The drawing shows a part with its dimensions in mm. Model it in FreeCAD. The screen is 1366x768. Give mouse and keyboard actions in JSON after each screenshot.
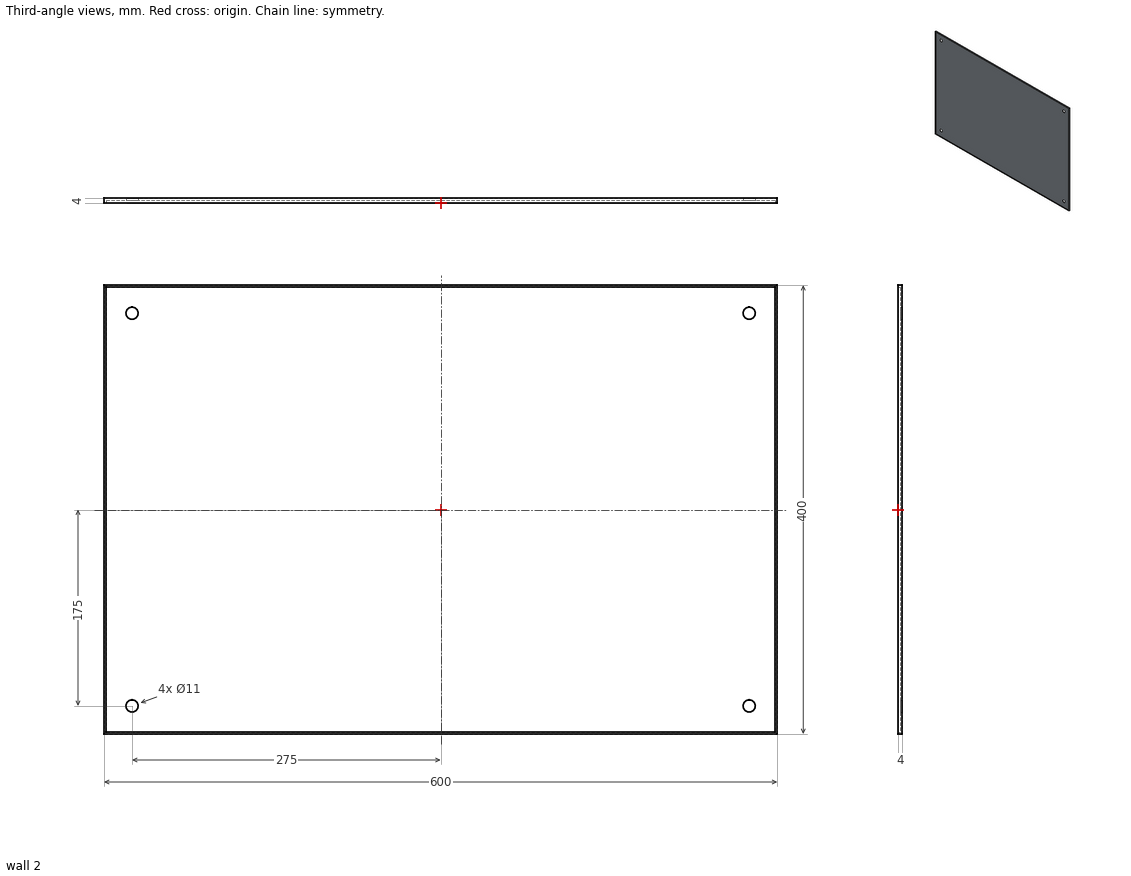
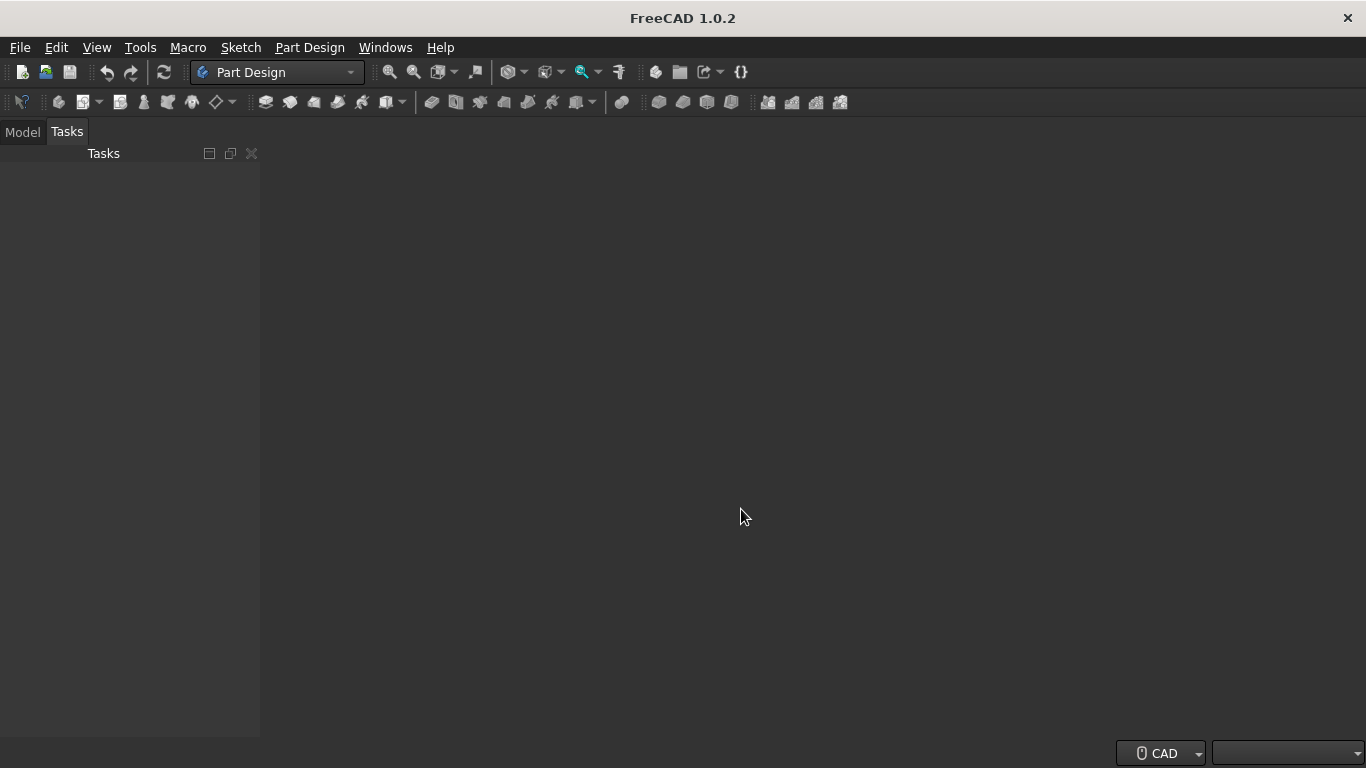
{"action": "key", "text": "ctrl+n"}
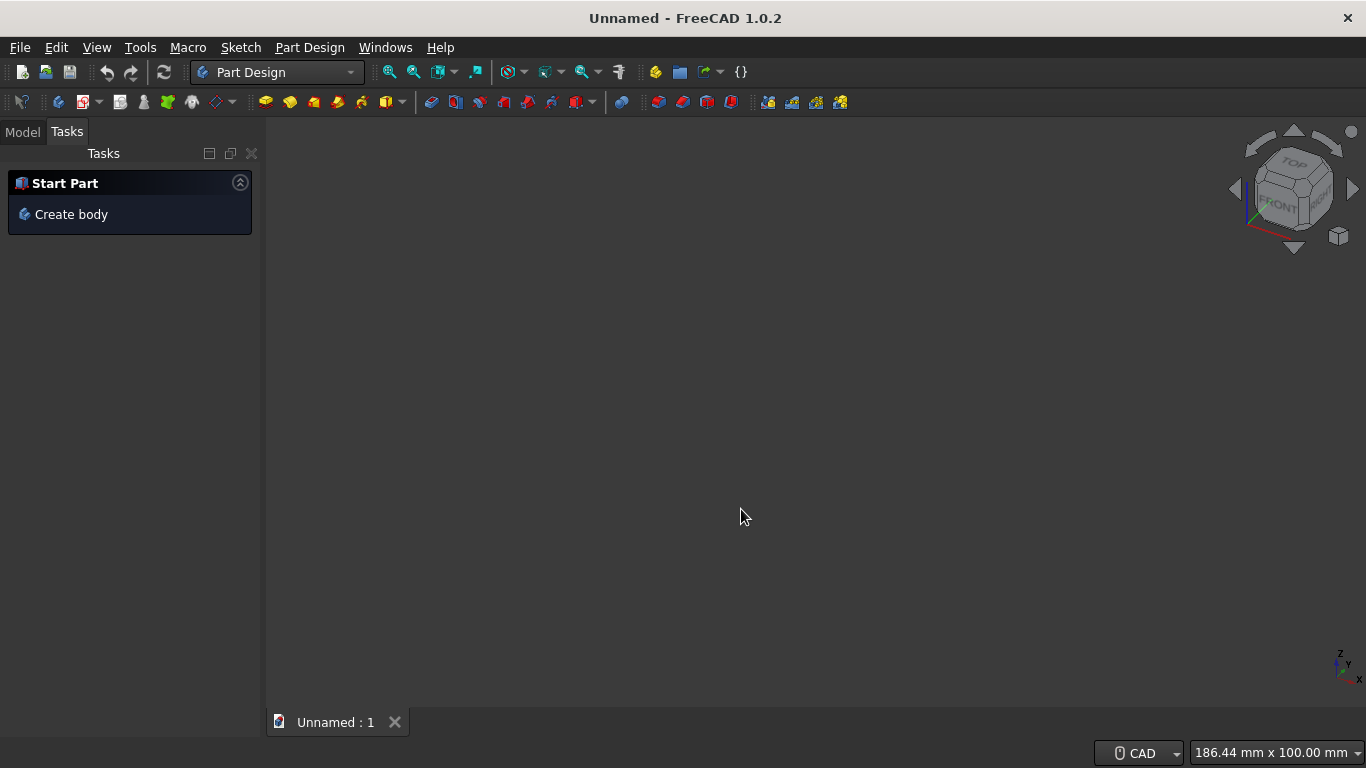
{"action": "left_click", "coordinate": [84, 102]}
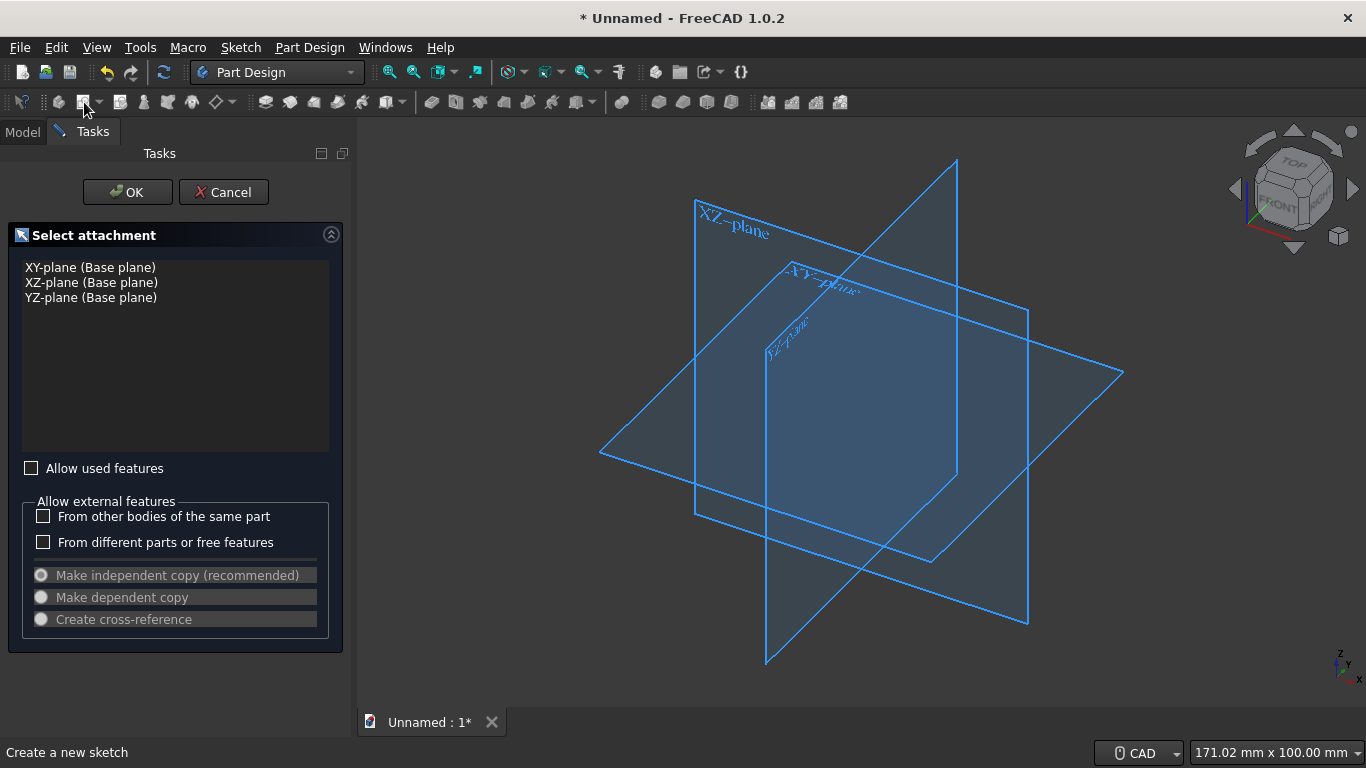
{"action": "left_click", "coordinate": [82, 282]}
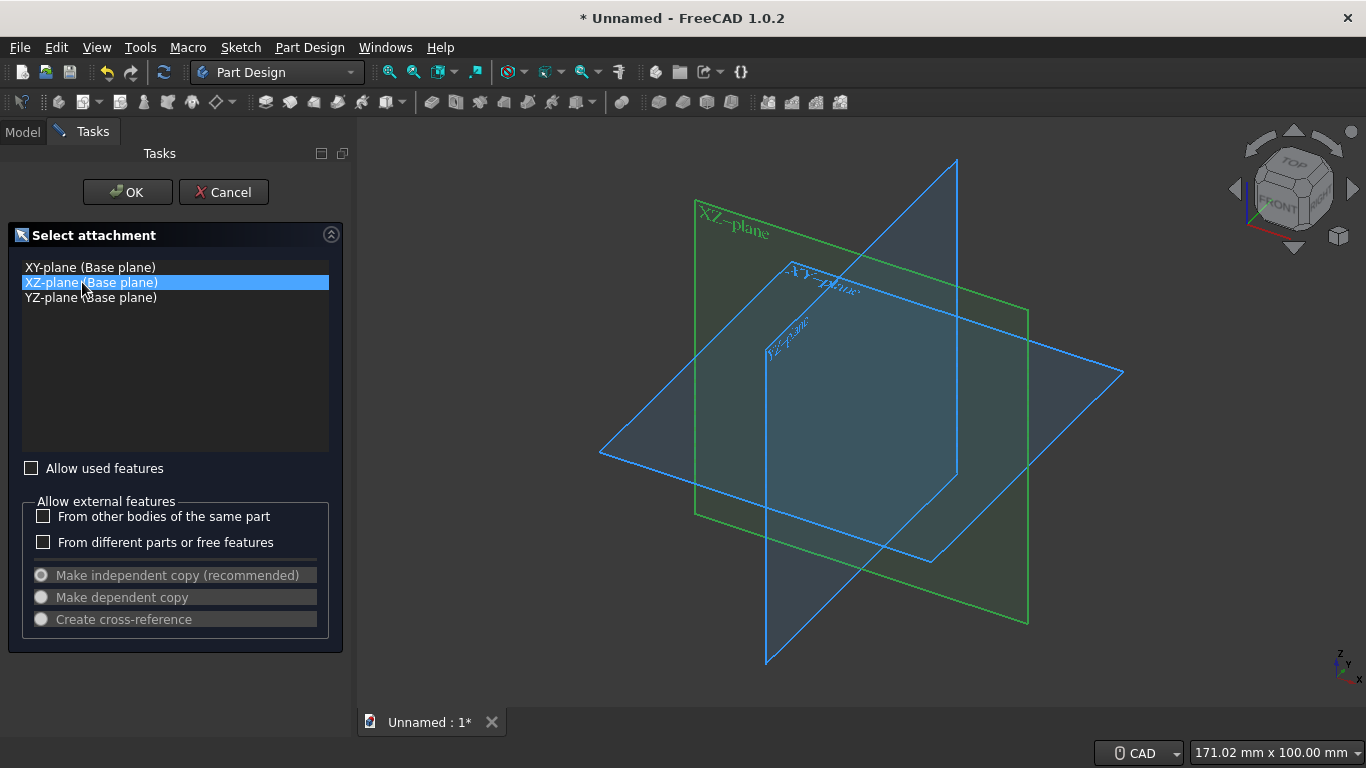
{"action": "left_click", "coordinate": [128, 192]}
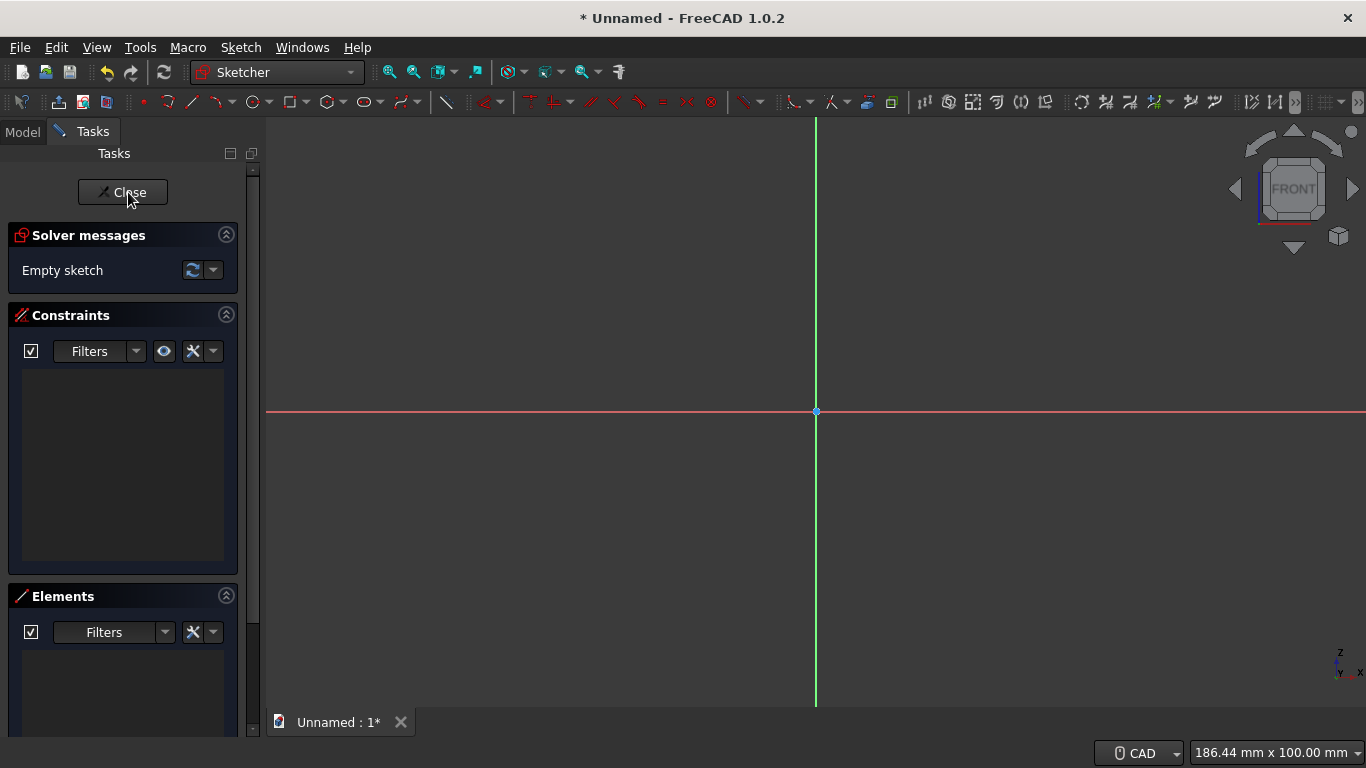
{"action": "scroll", "coordinate": [734, 412], "scroll_direction": "down", "scroll_amount": 9}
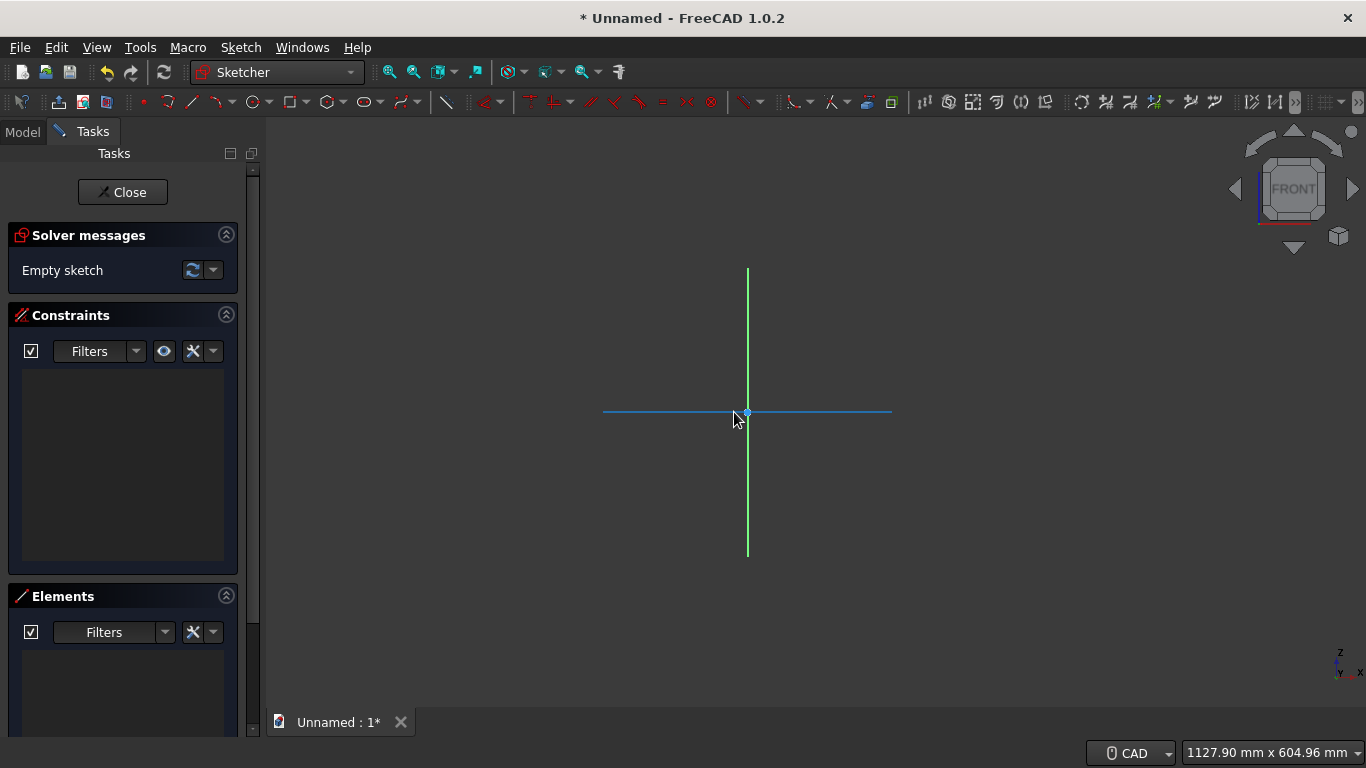
{"action": "key", "text": "g v"}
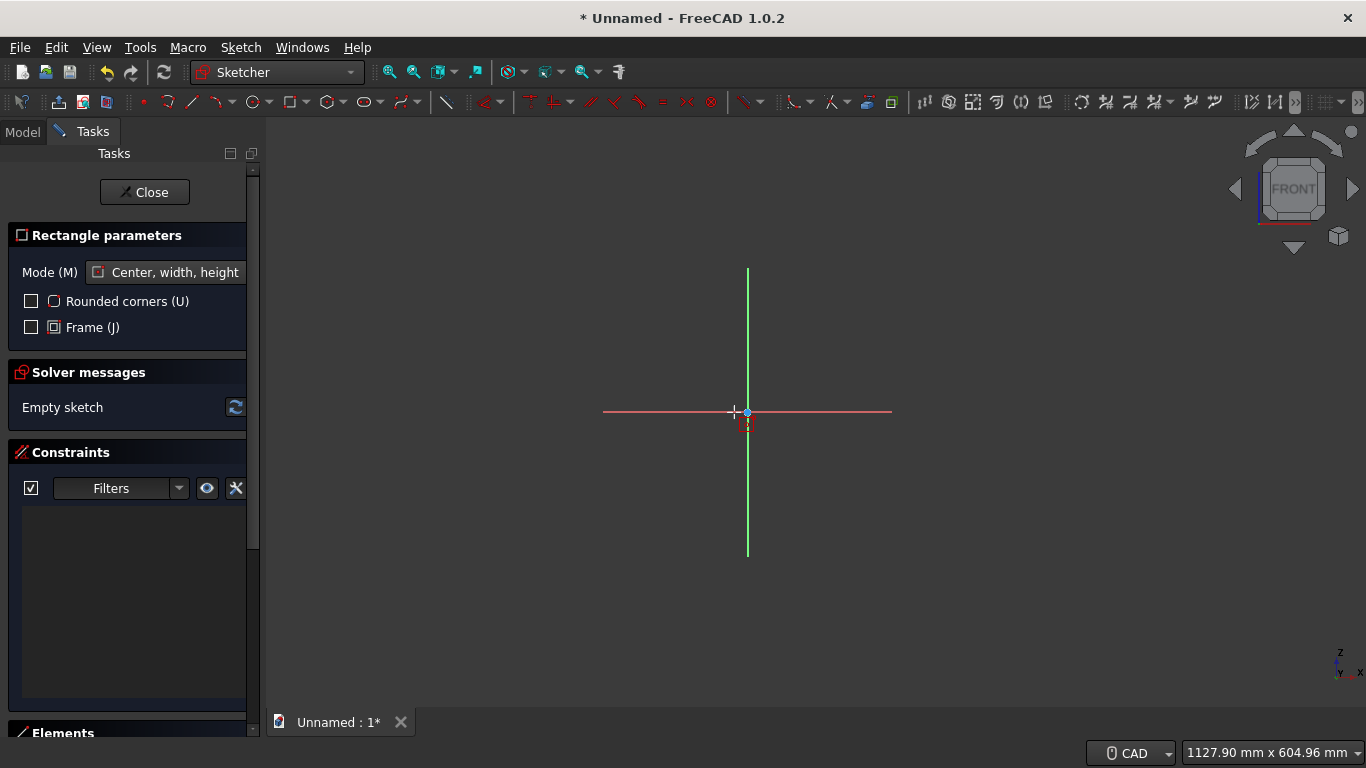
{"action": "left_click", "coordinate": [748, 412]}
{"action": "left_click", "coordinate": [1040, 217]}
{"action": "key", "text": "Escape"}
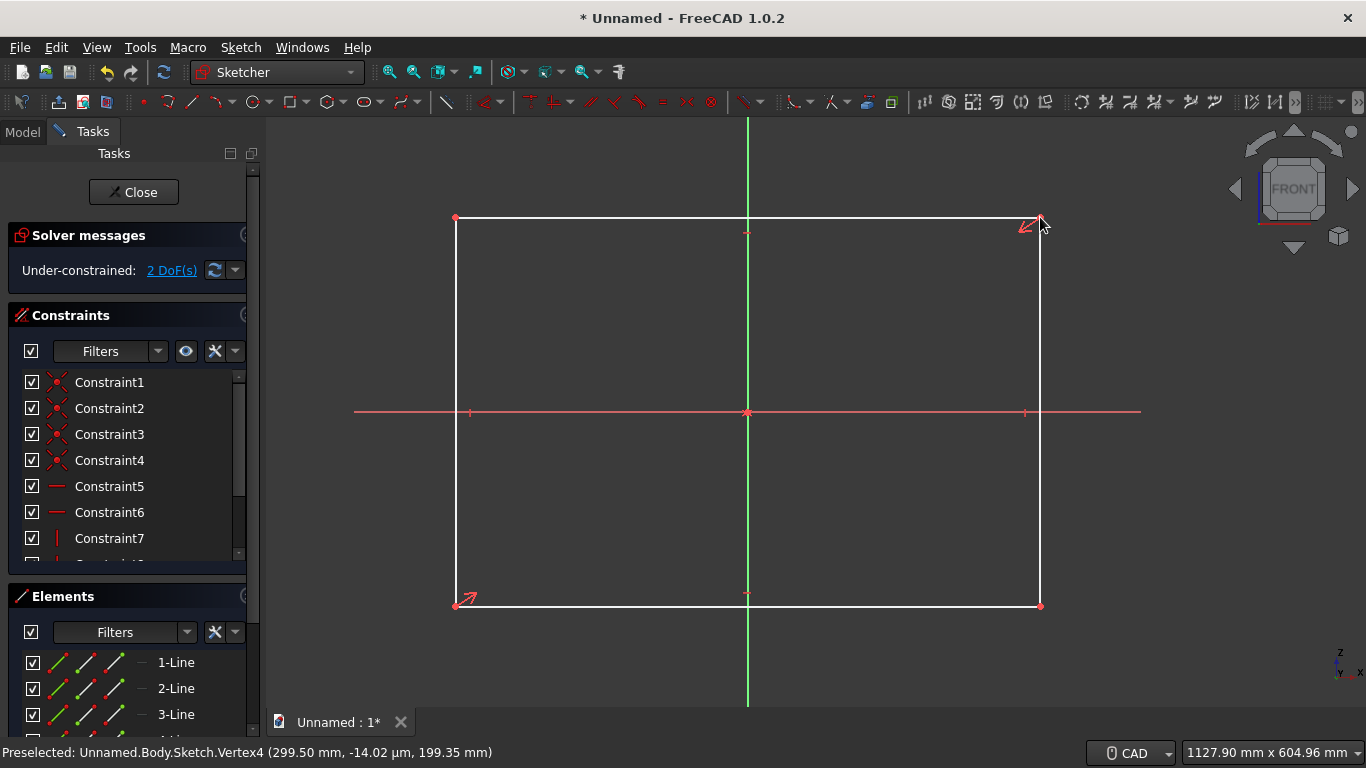
{"action": "key", "text": "d"}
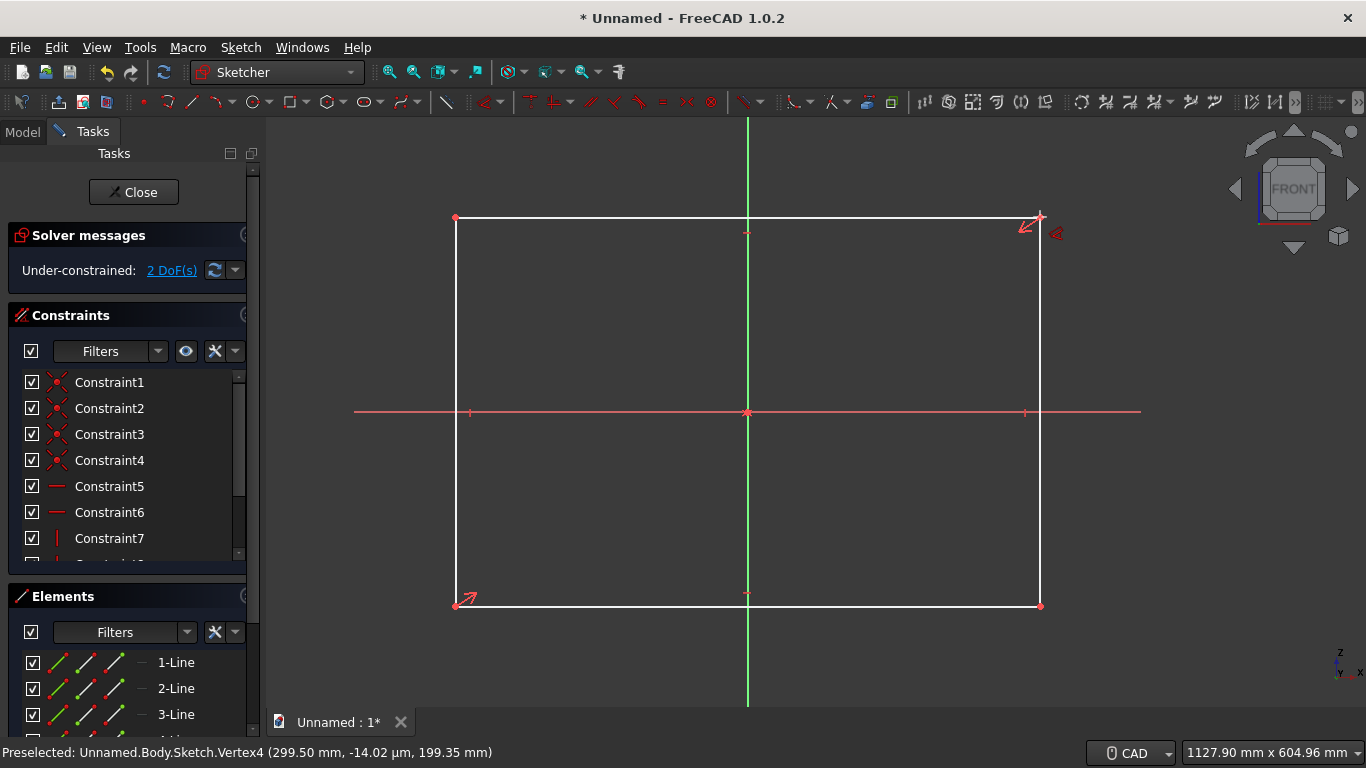
{"action": "left_click", "coordinate": [631, 607]}
{"action": "left_click", "coordinate": [614, 641]}